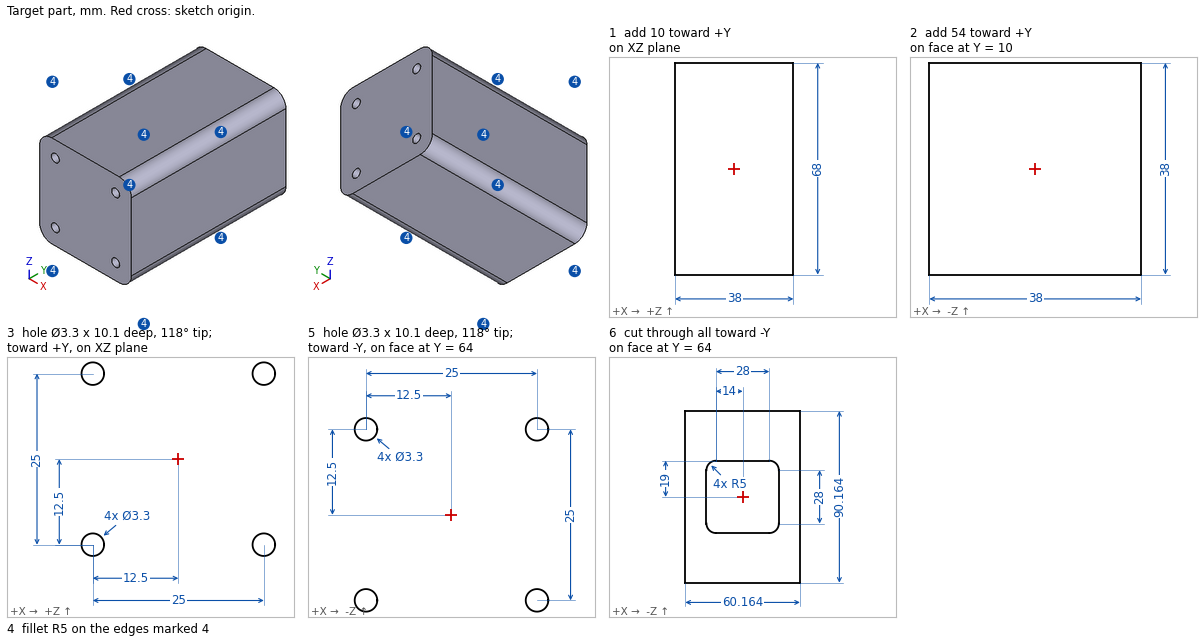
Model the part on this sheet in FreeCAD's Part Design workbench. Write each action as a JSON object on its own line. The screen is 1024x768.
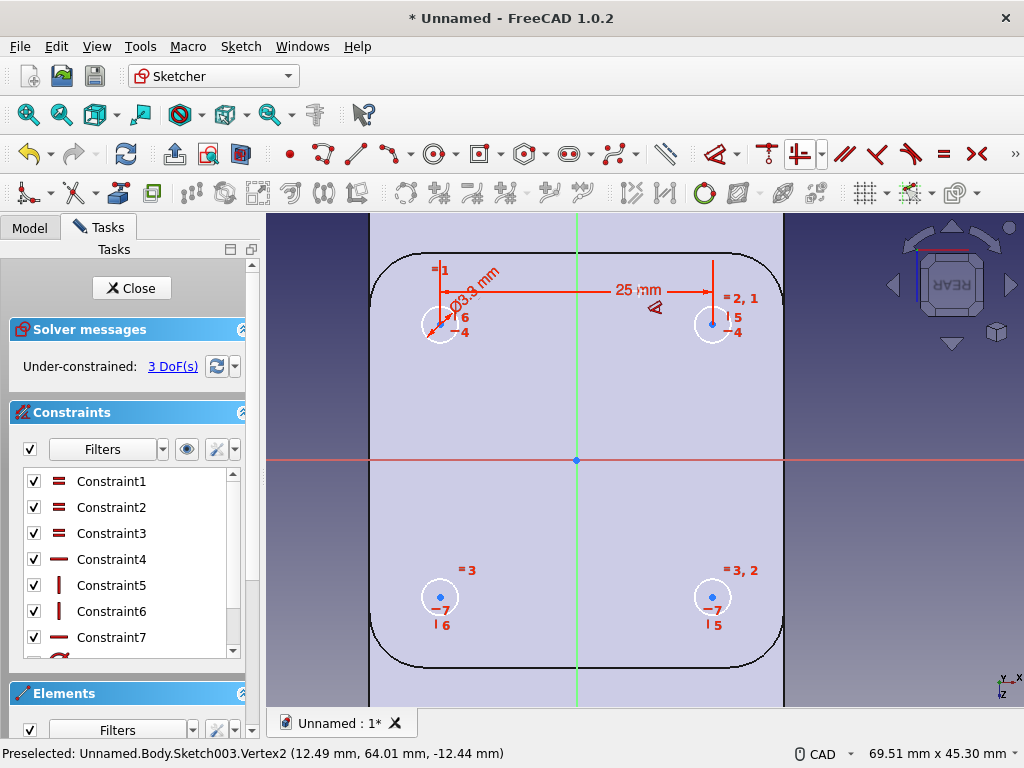
{"action": "left_click", "coordinate": [713, 325]}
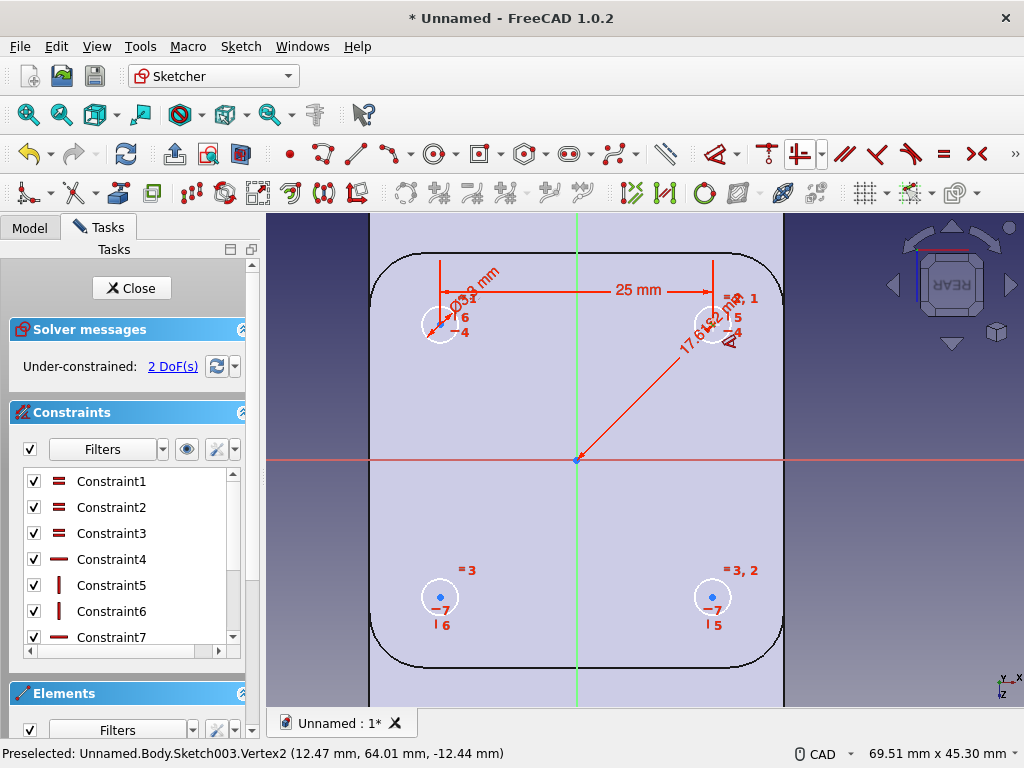
{"action": "left_click", "coordinate": [713, 597]}
{"action": "left_click", "coordinate": [747, 398]}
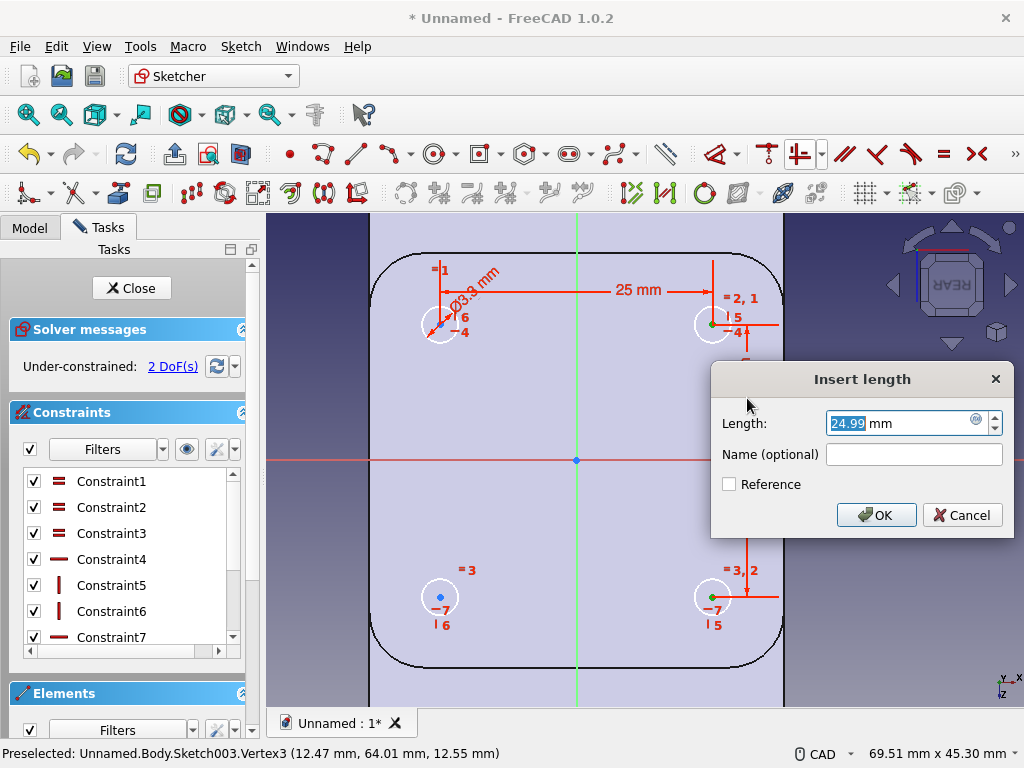
{"action": "type", "text": "25"}
{"action": "key", "text": "Return"}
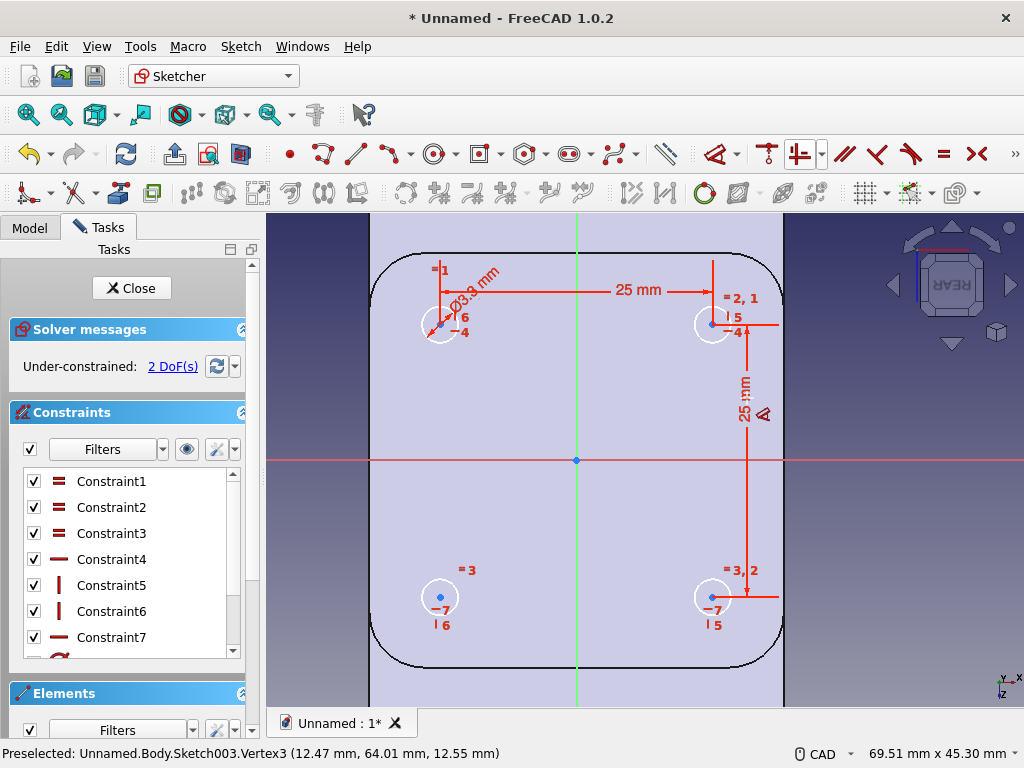
{"action": "left_click", "coordinate": [440, 325]}
{"action": "left_click", "coordinate": [556, 291]}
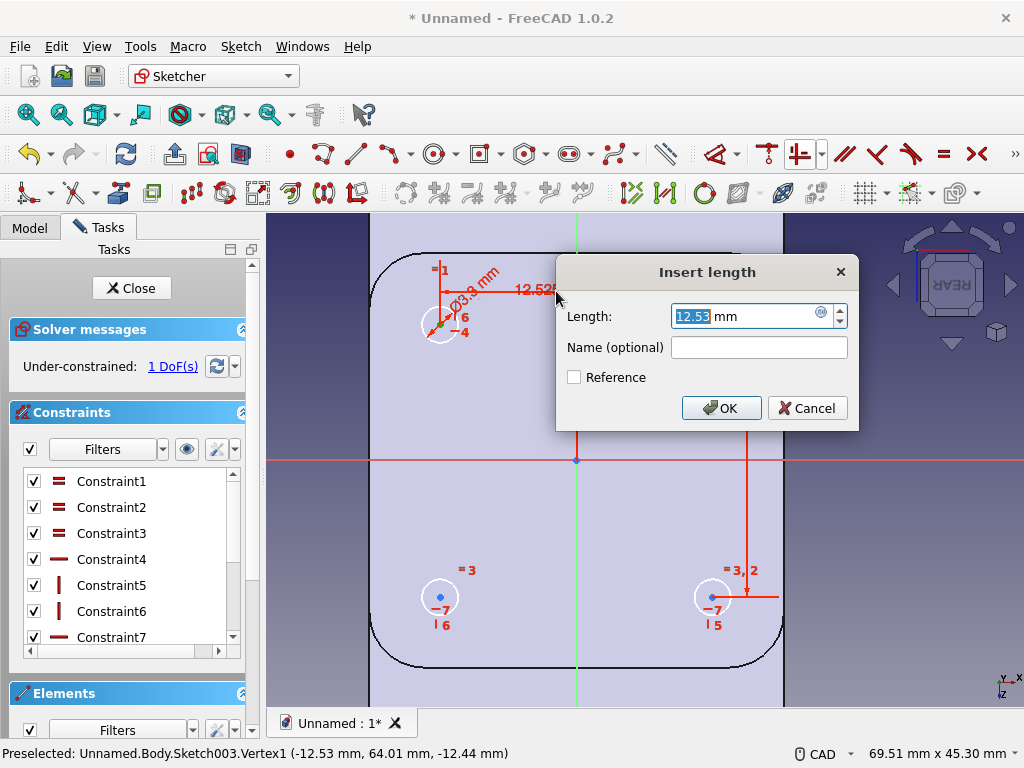
{"action": "type", "text": "12.5"}
{"action": "key", "text": "Return"}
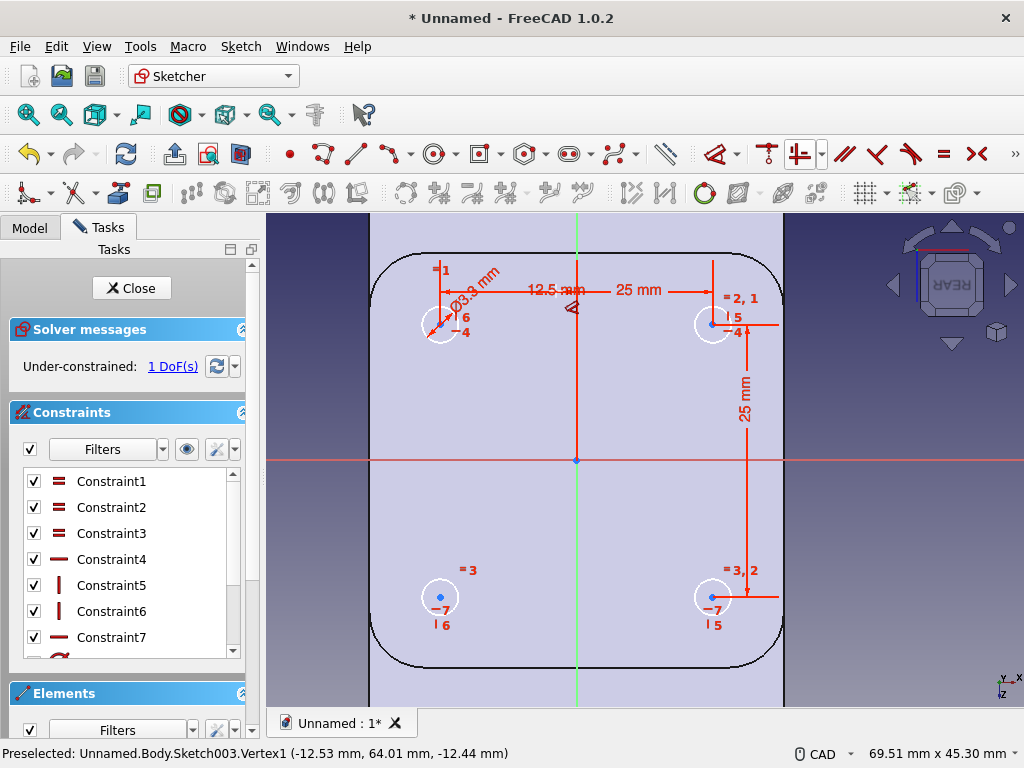
{"action": "left_click", "coordinate": [440, 325]}
{"action": "left_click", "coordinate": [406, 393]}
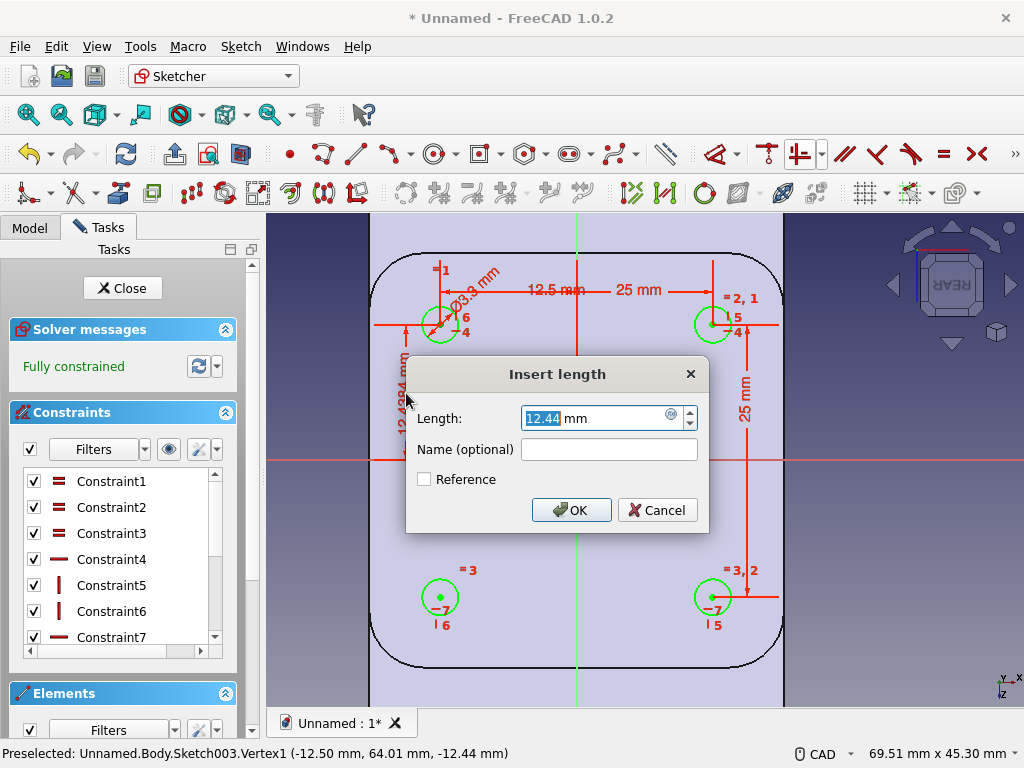
{"action": "type", "text": "12.5"}
{"action": "key", "text": "Return"}
{"action": "key", "text": "Escape"}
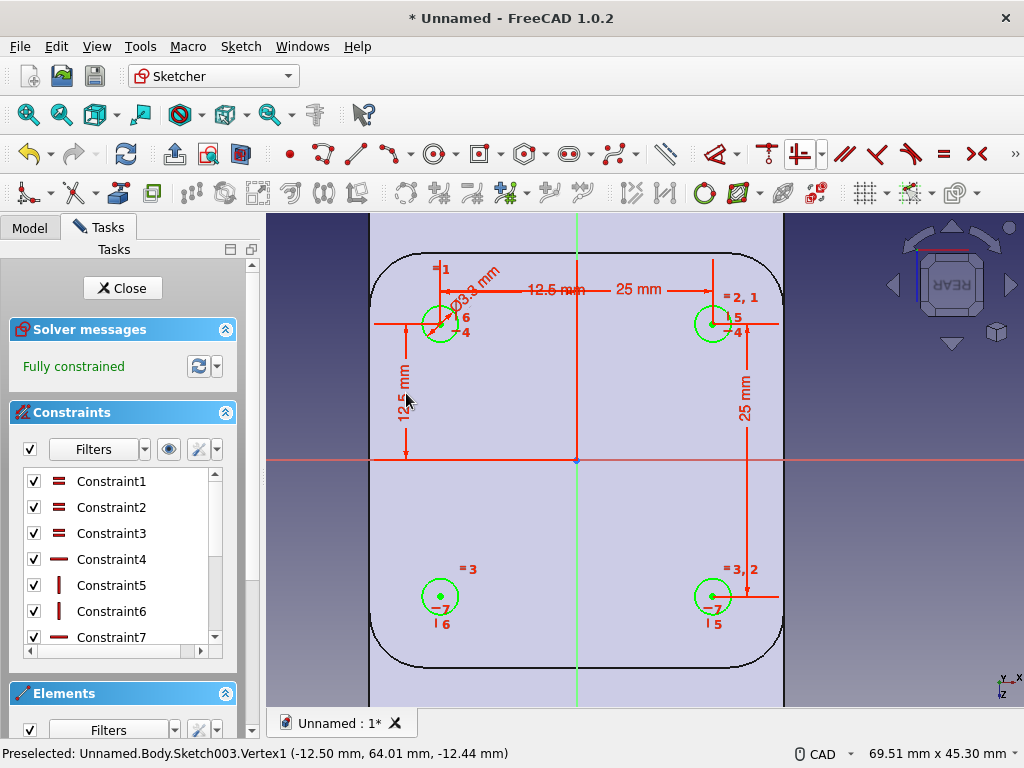
{"action": "left_click", "coordinate": [123, 288]}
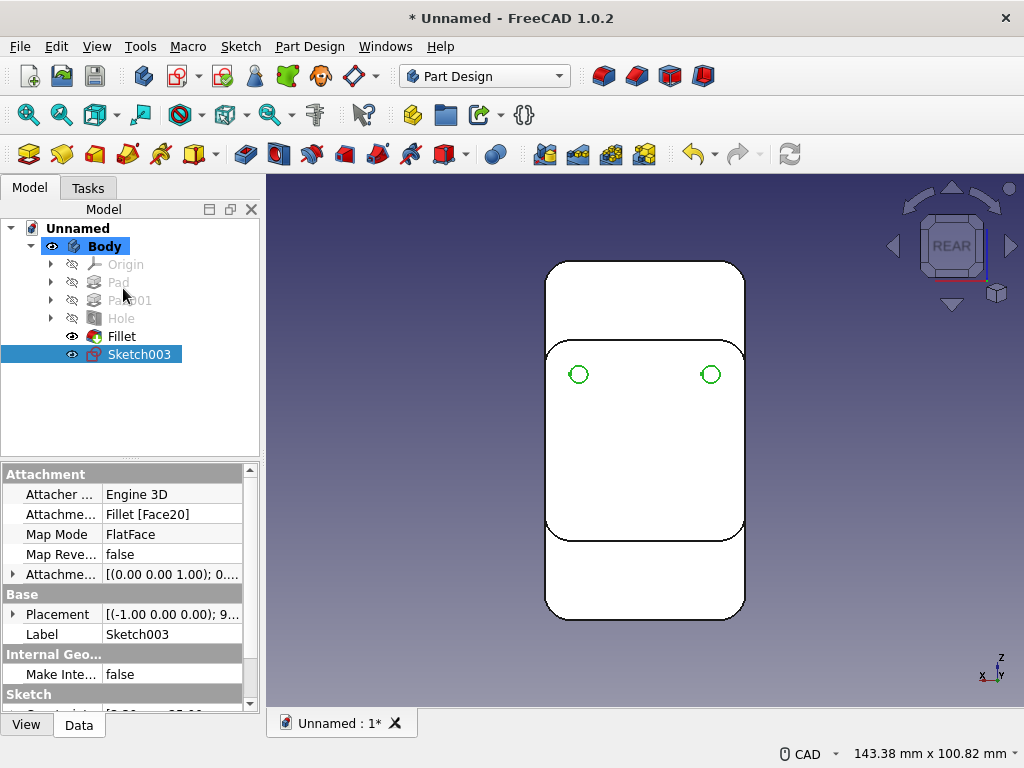
{"action": "left_click", "coordinate": [279, 154]}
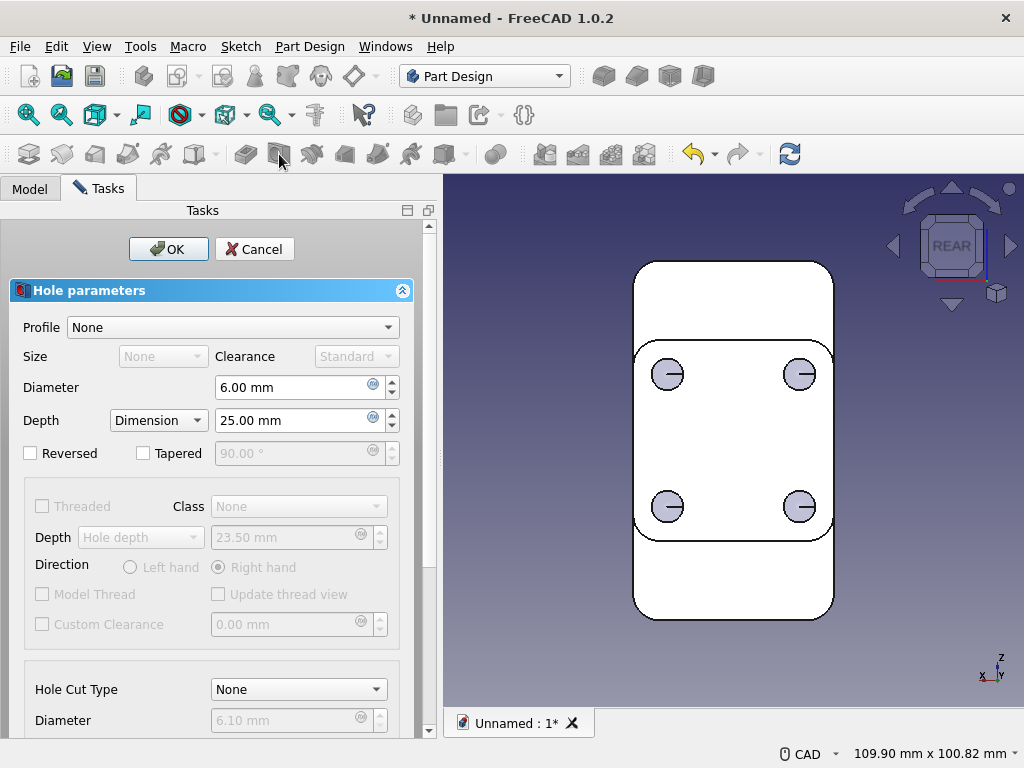
{"action": "triple_click", "coordinate": [300, 388]}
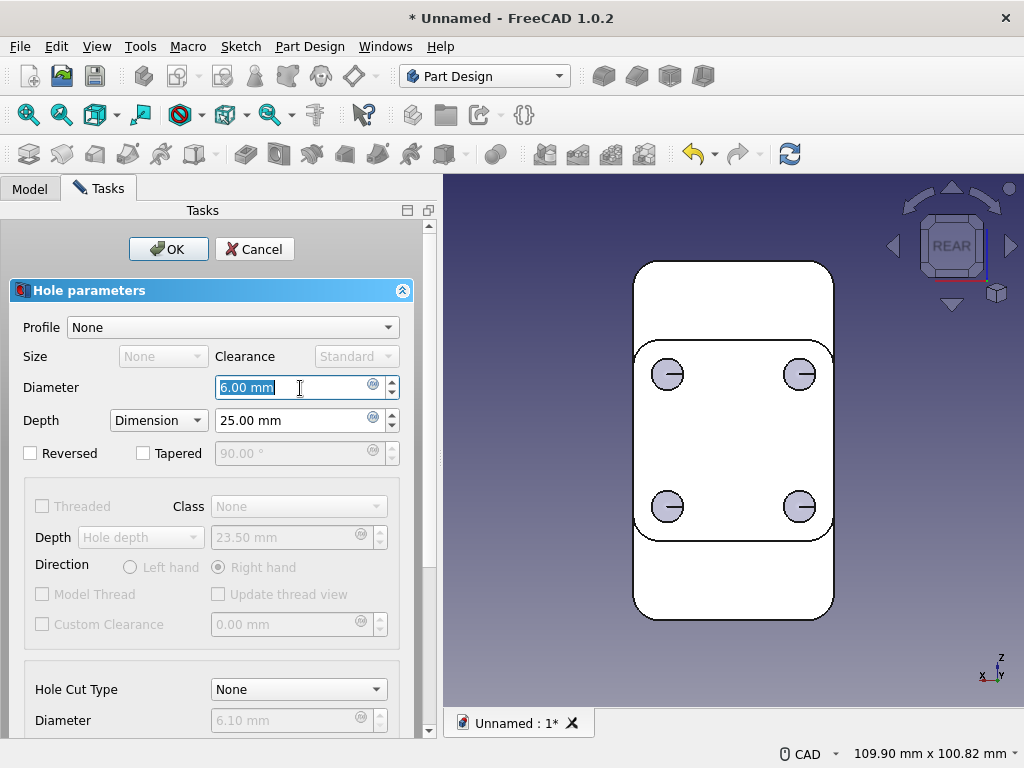
{"action": "type", "text": "3.3"}
{"action": "key", "text": "Tab"}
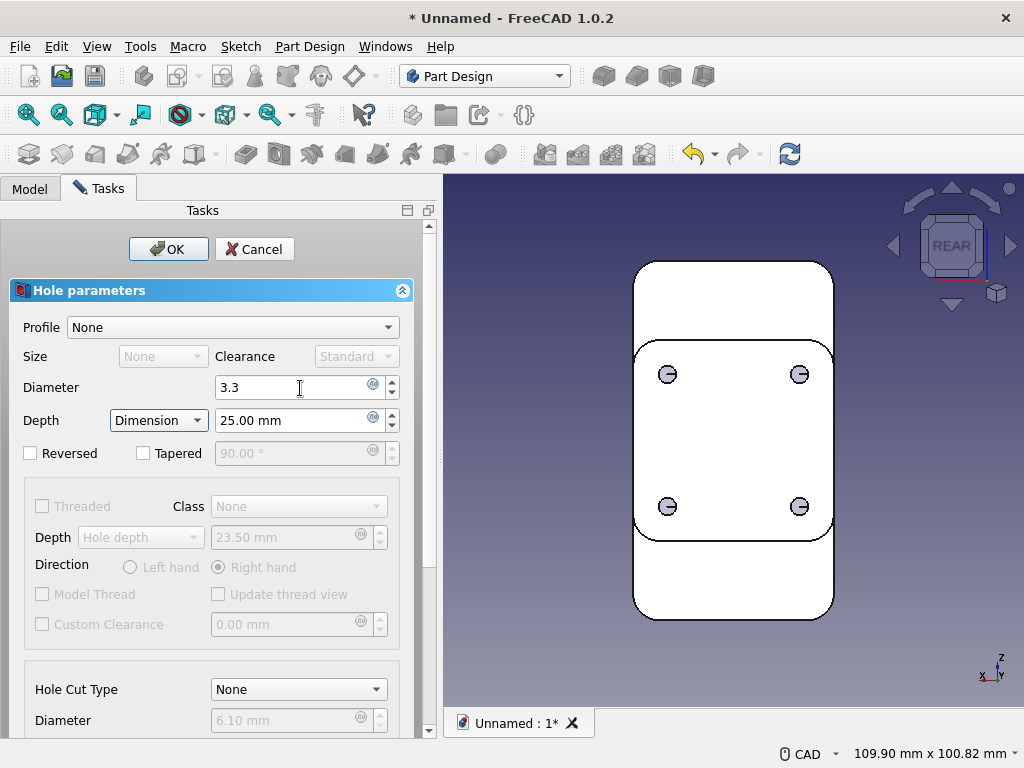
{"action": "triple_click", "coordinate": [300, 420]}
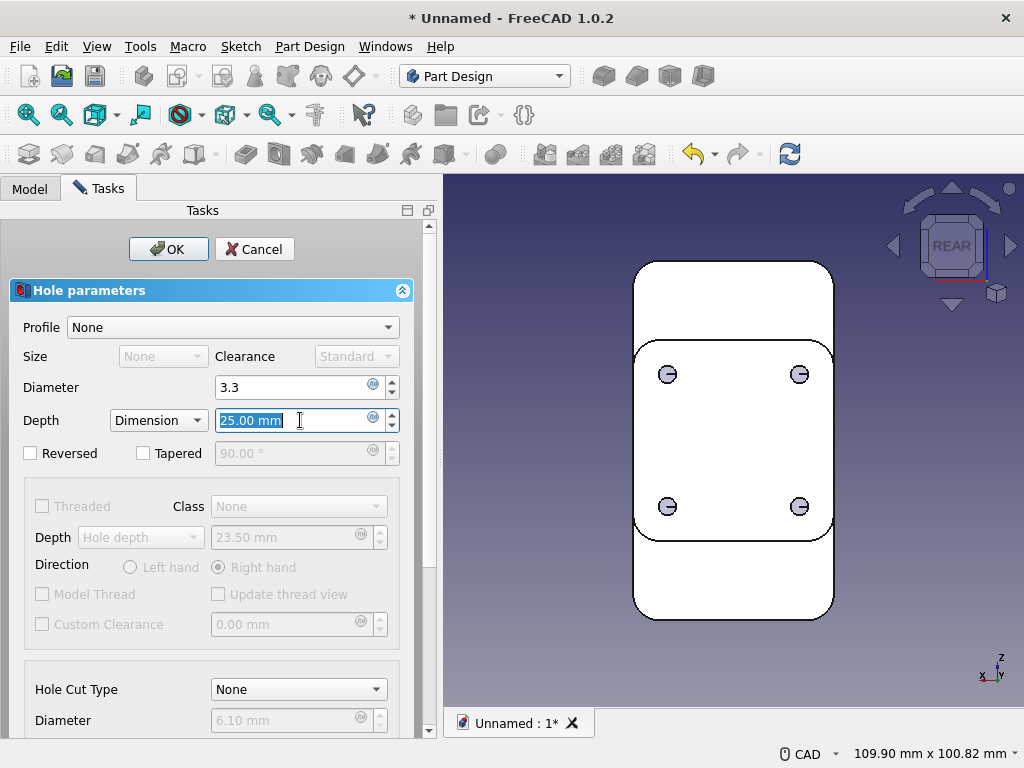
{"action": "type", "text": "10.1"}
{"action": "key", "text": "Tab"}